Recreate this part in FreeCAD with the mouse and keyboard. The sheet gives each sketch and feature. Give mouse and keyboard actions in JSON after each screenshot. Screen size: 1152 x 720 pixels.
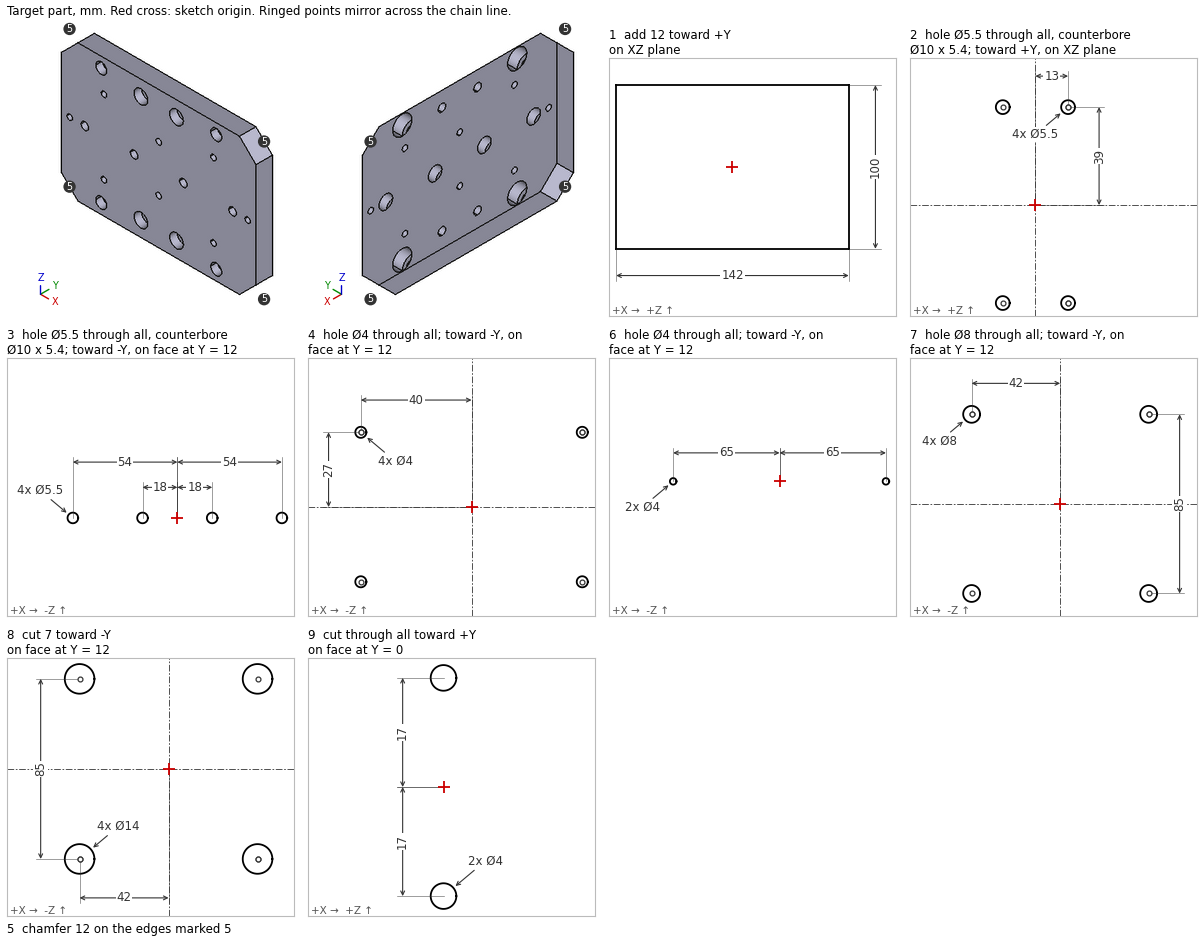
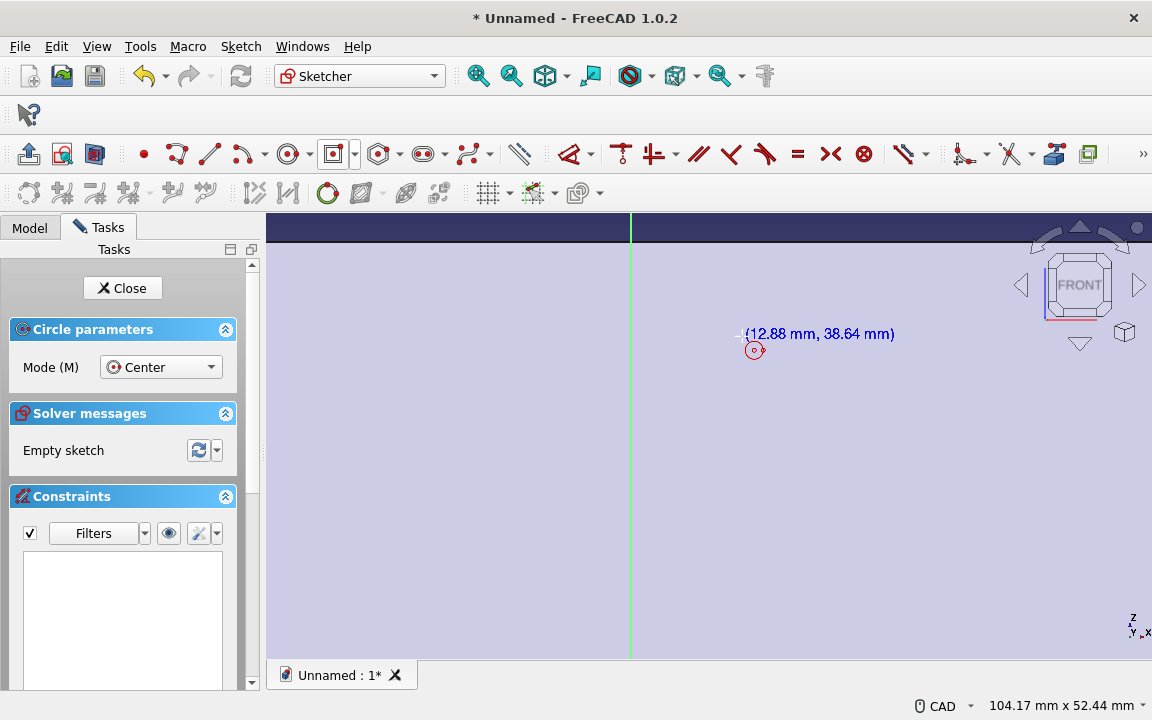
{"action": "left_click", "coordinate": [742, 336]}
{"action": "left_click", "coordinate": [758, 319]}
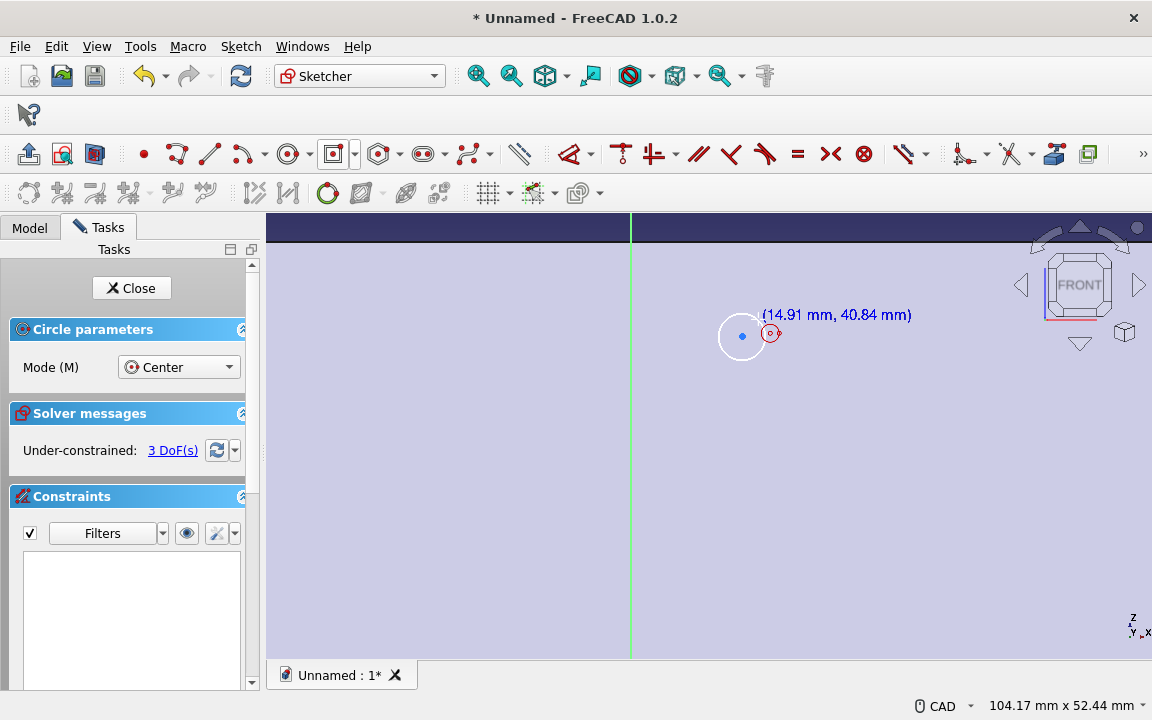
{"action": "scroll", "coordinate": [646, 301], "scroll_direction": "down", "scroll_amount": 5}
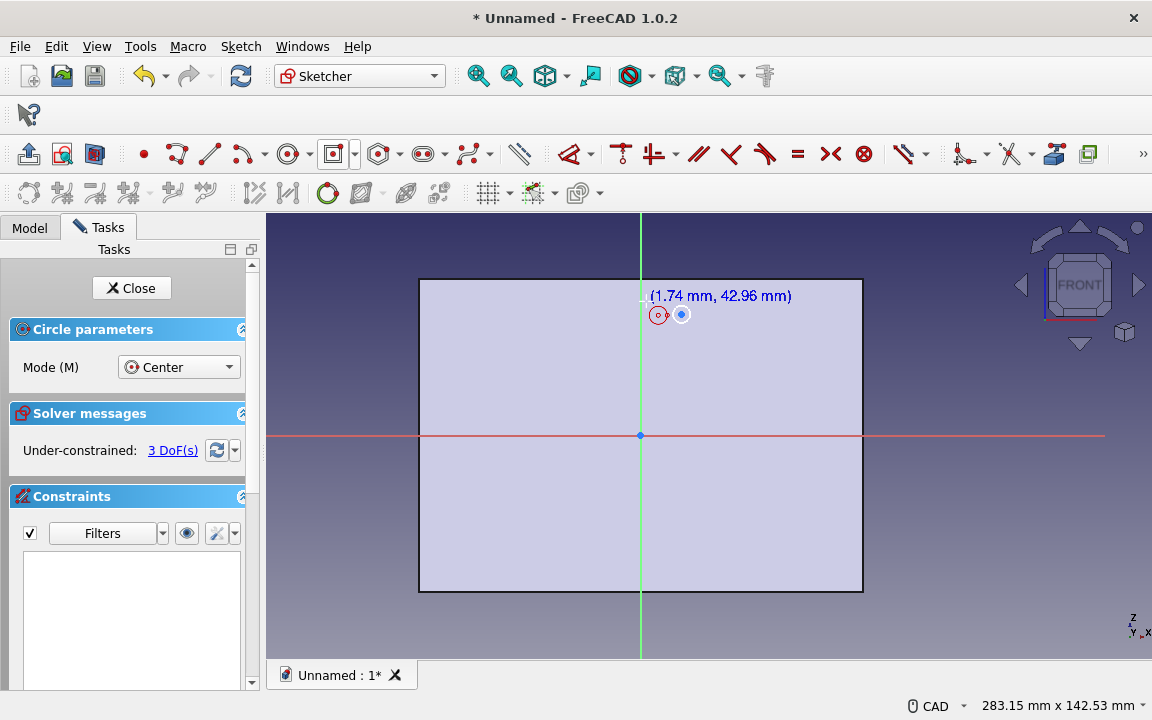
{"action": "scroll", "coordinate": [600, 558], "scroll_direction": "up", "scroll_amount": 5}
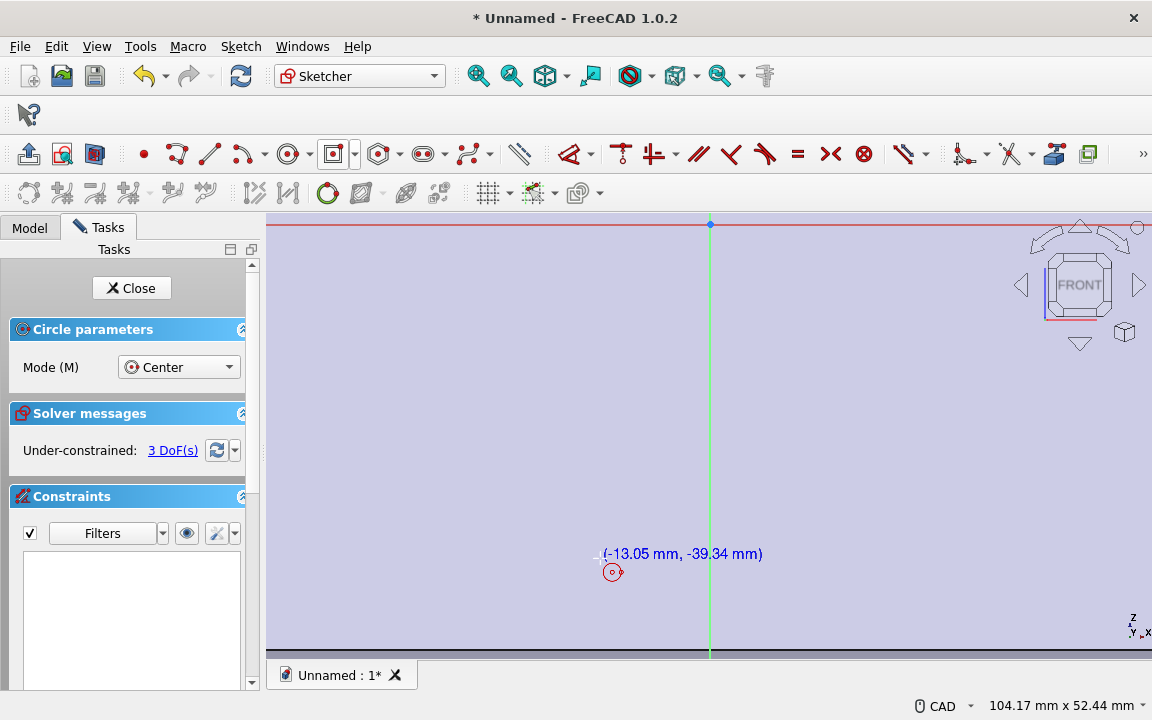
{"action": "left_click", "coordinate": [600, 557]}
{"action": "left_click", "coordinate": [616, 540]}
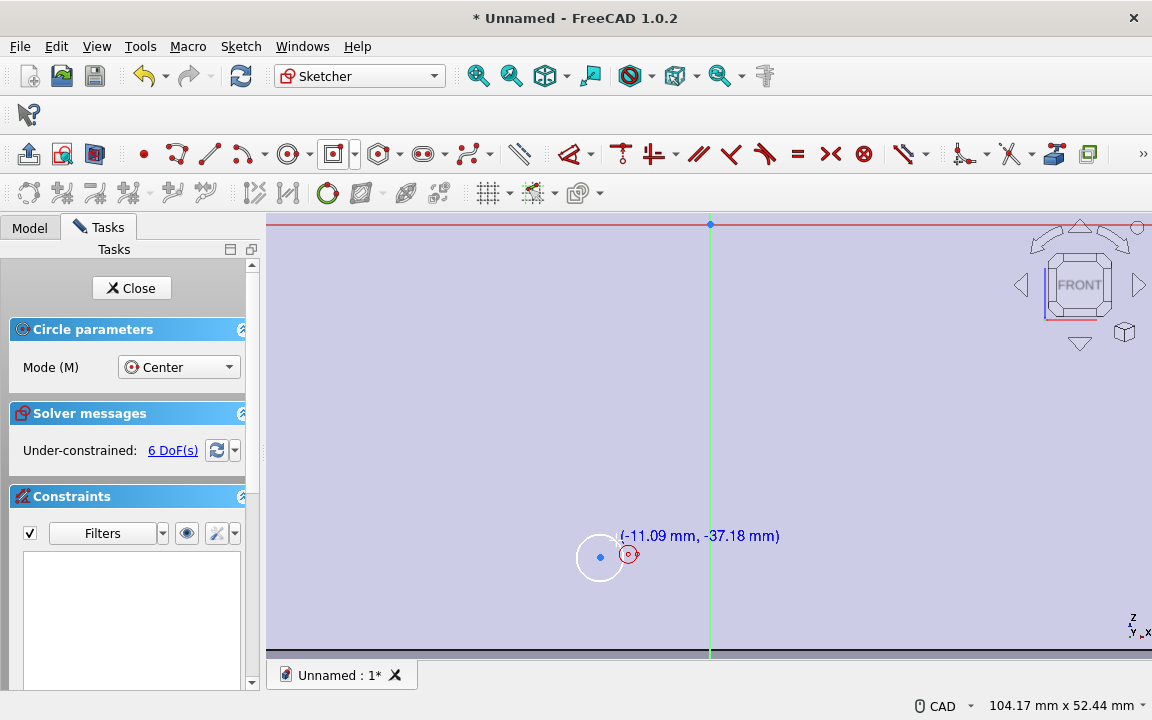
{"action": "left_click", "coordinate": [821, 557]}
{"action": "left_click", "coordinate": [837, 540]}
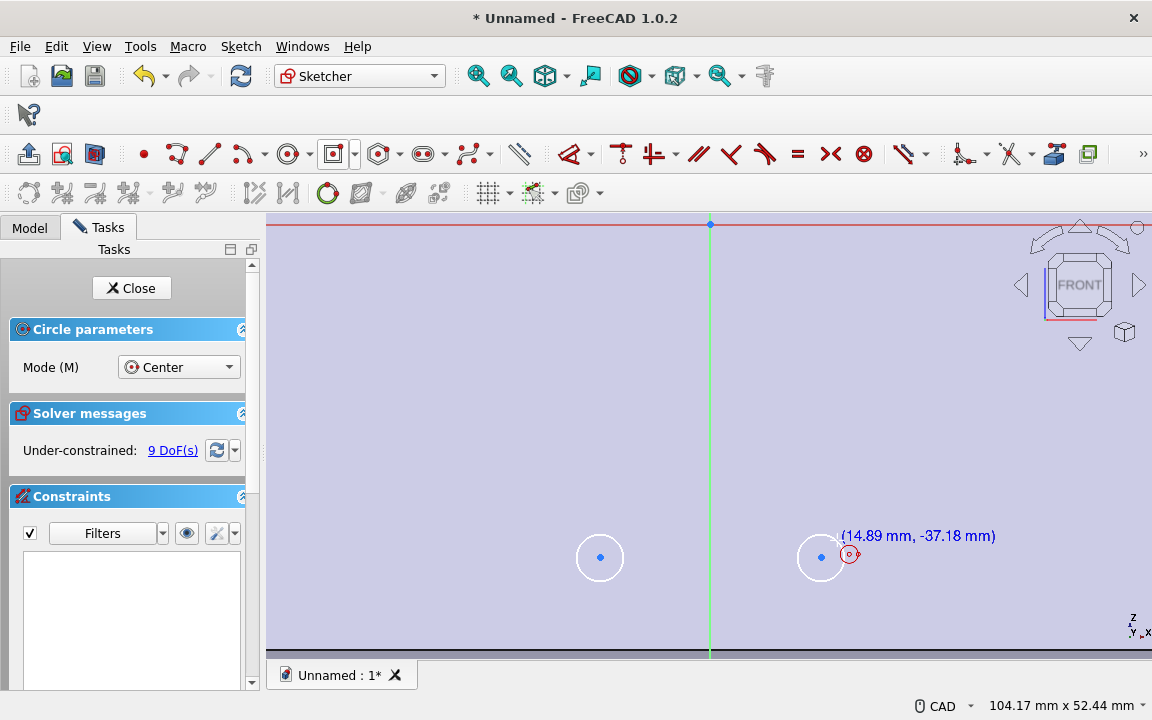
{"action": "scroll", "coordinate": [600, 559], "scroll_direction": "down", "scroll_amount": 5}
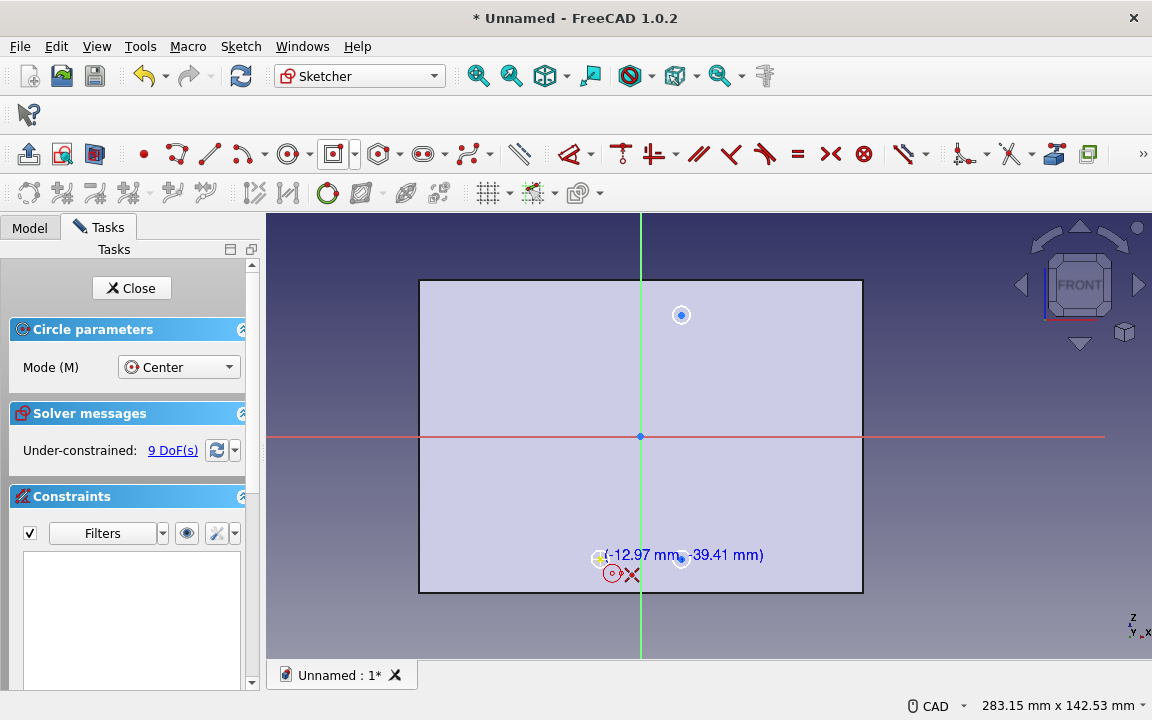
{"action": "scroll", "coordinate": [600, 315], "scroll_direction": "up", "scroll_amount": 5}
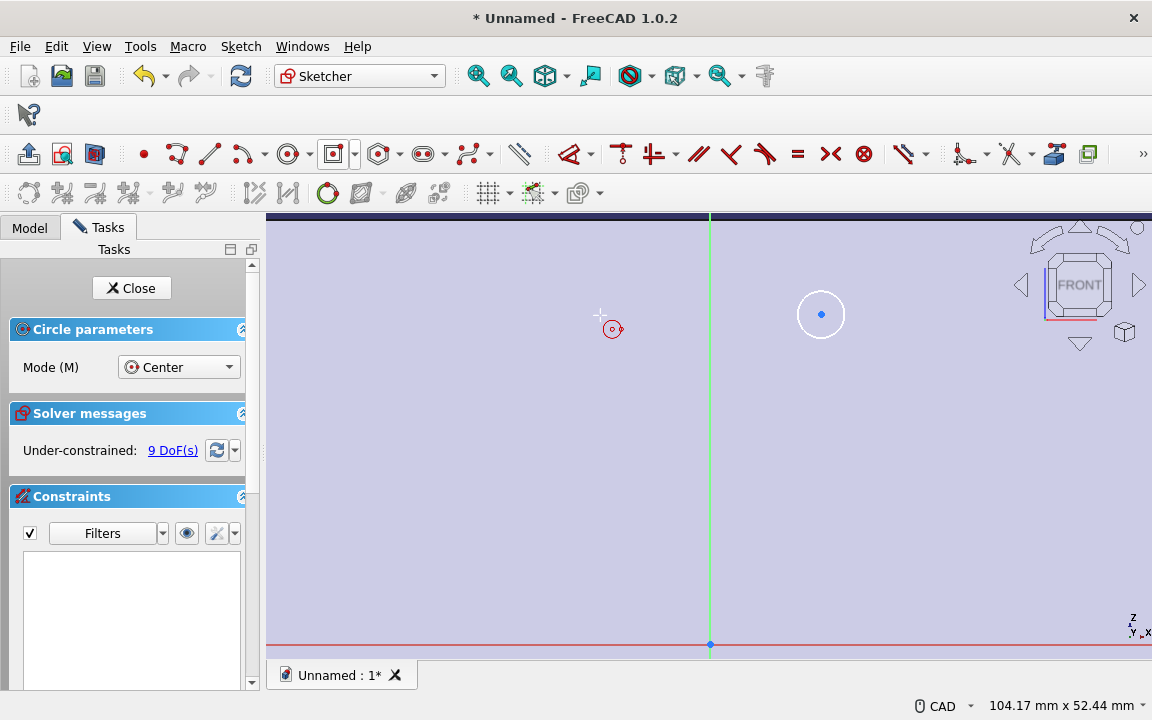
{"action": "left_click", "coordinate": [600, 313]}
{"action": "left_click", "coordinate": [616, 297]}
{"action": "key", "text": "Escape"}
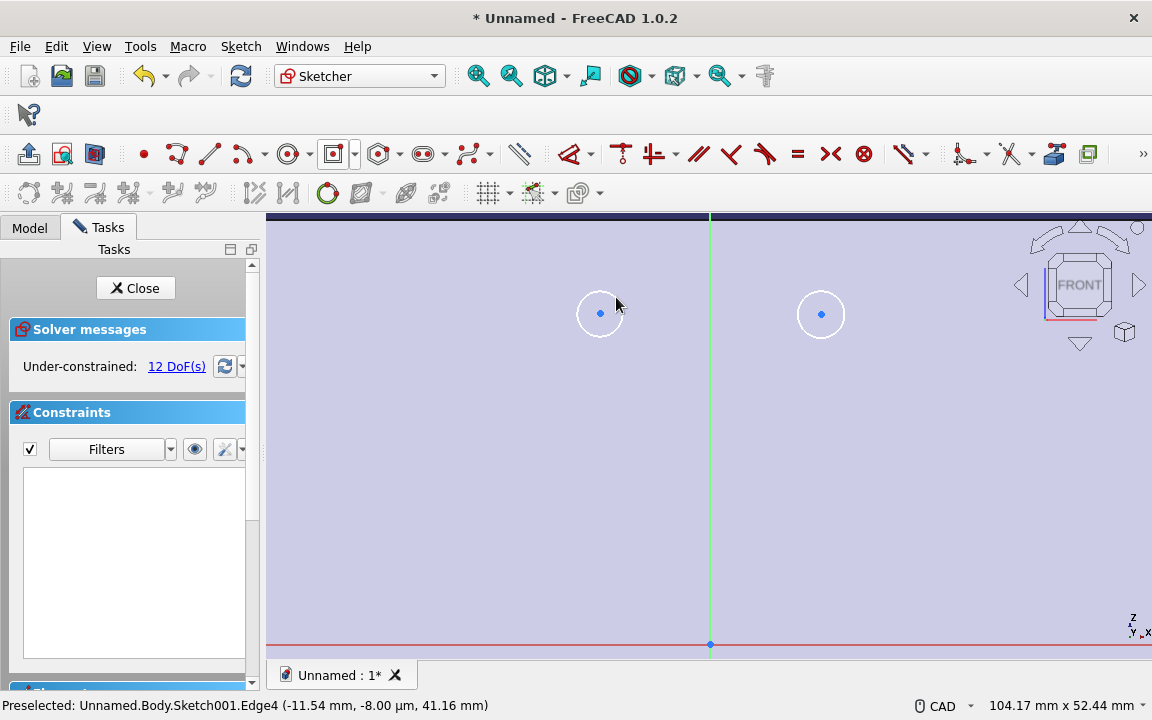
{"action": "left_click", "coordinate": [838, 298]}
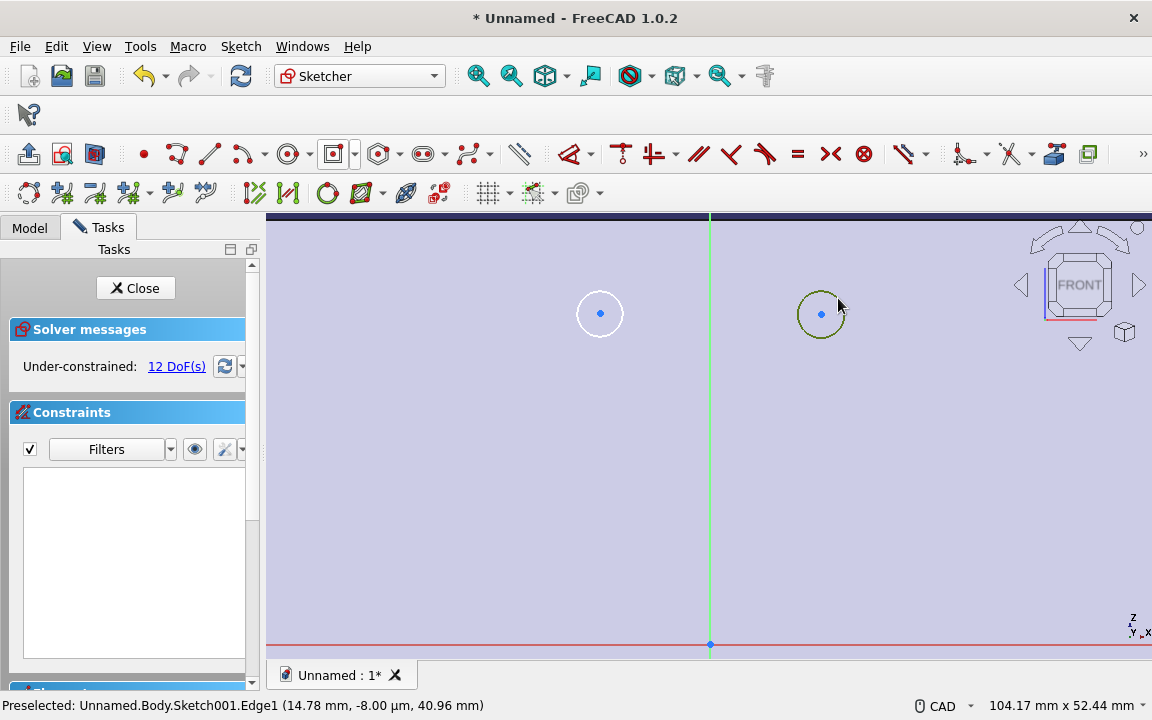
{"action": "scroll", "coordinate": [600, 314], "scroll_direction": "down", "scroll_amount": 5}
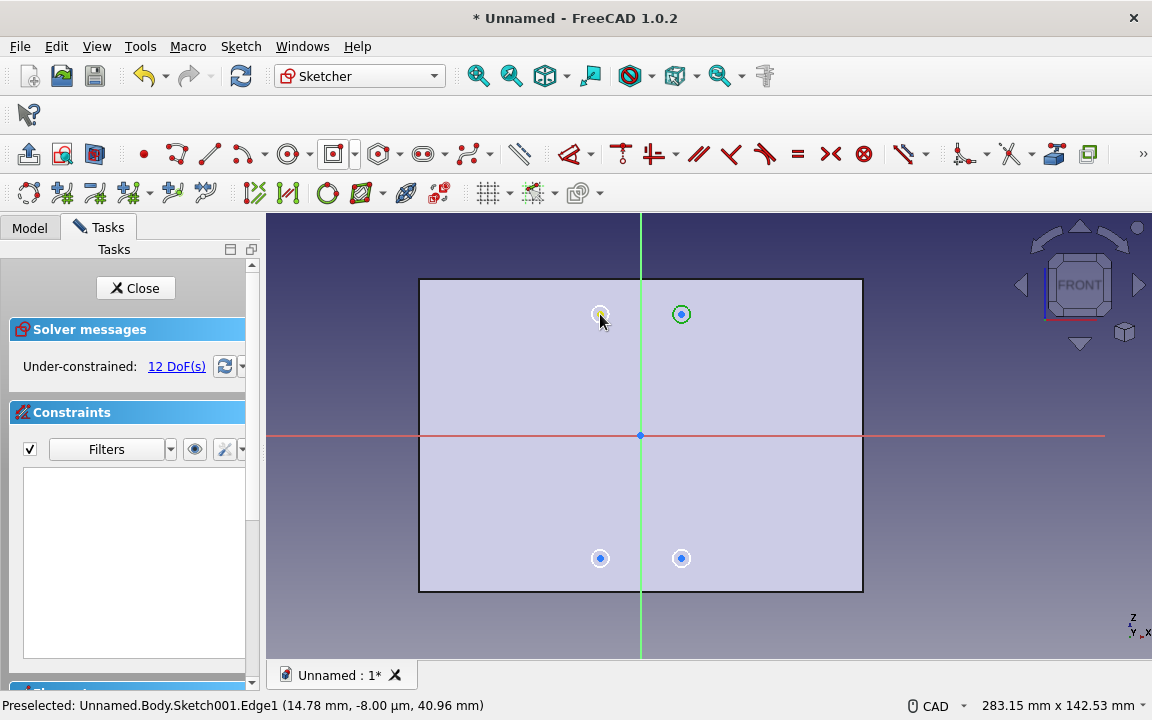
{"action": "scroll", "coordinate": [606, 552], "scroll_direction": "up", "scroll_amount": 3}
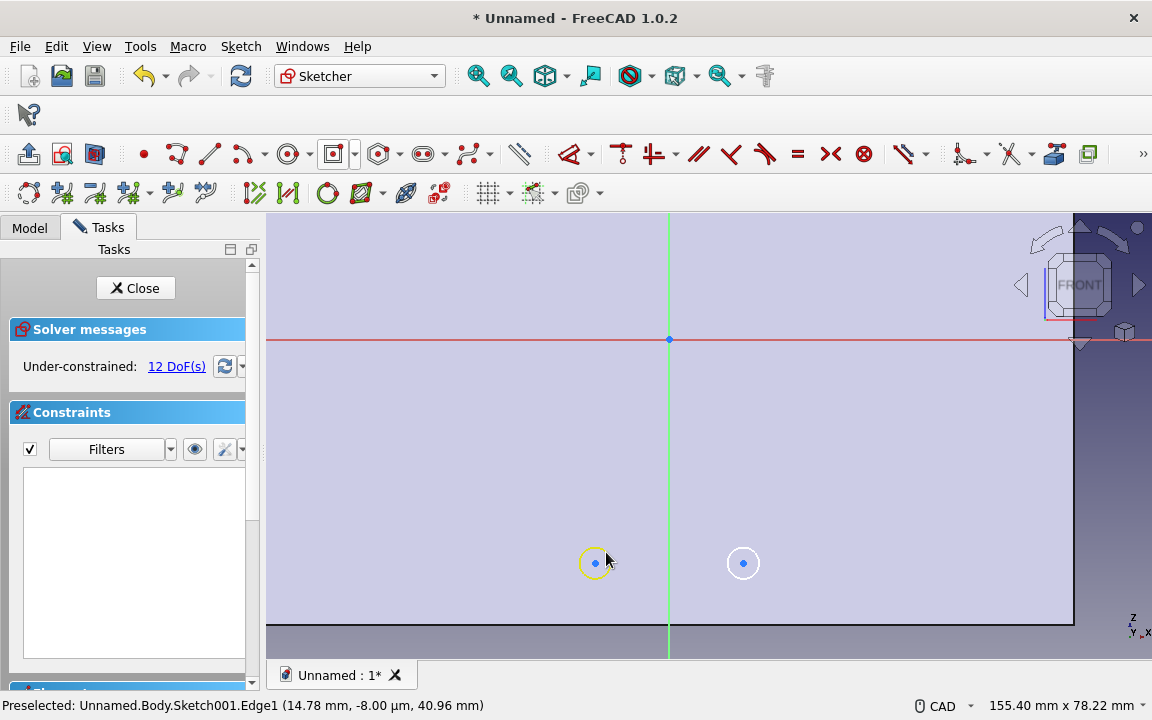
{"action": "left_click", "coordinate": [606, 552]}